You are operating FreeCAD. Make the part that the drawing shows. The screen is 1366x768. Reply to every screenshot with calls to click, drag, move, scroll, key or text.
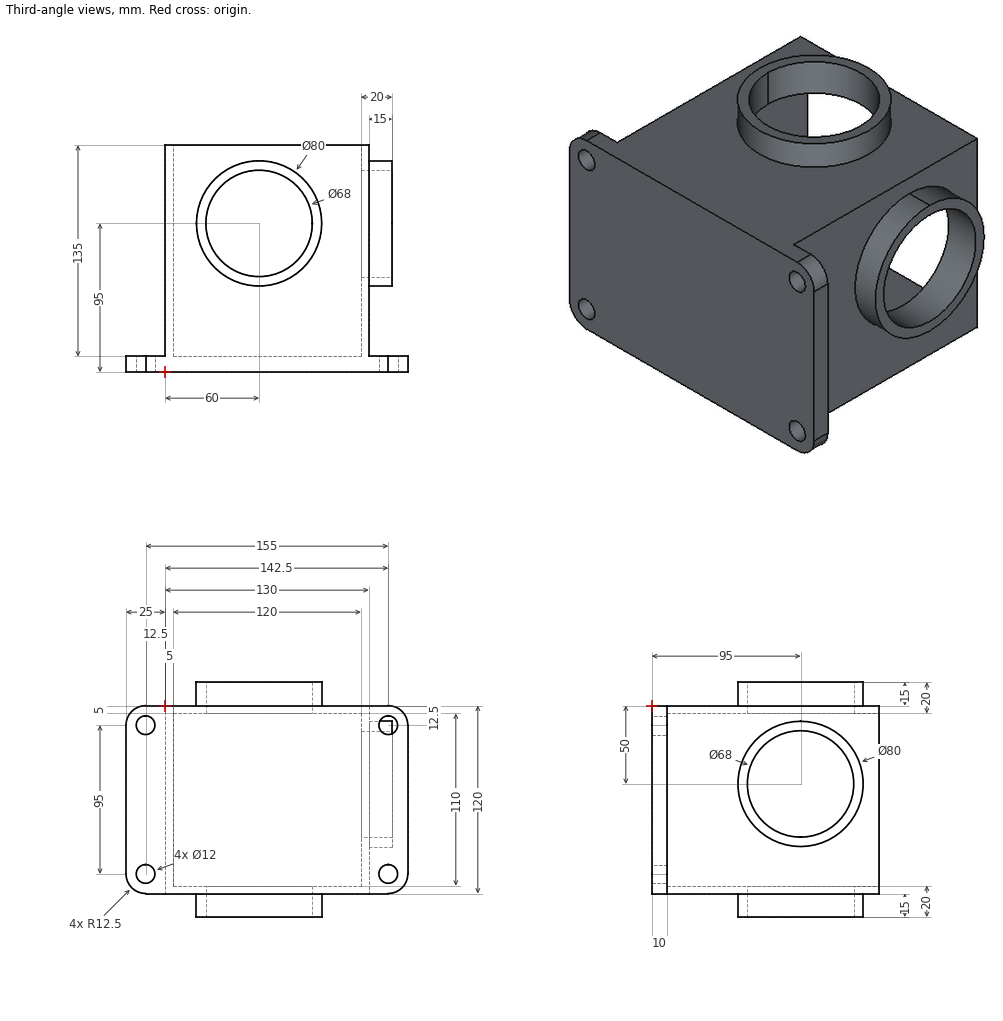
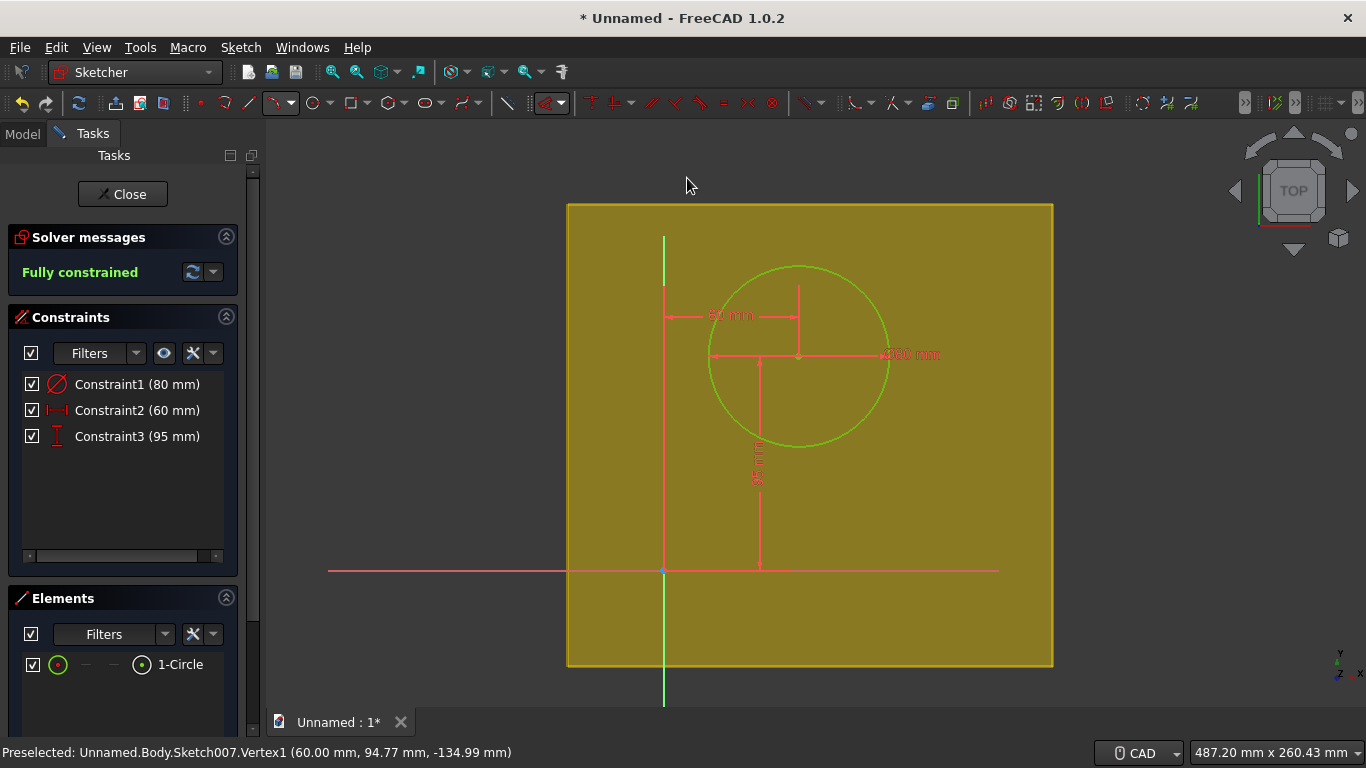
click(123, 194)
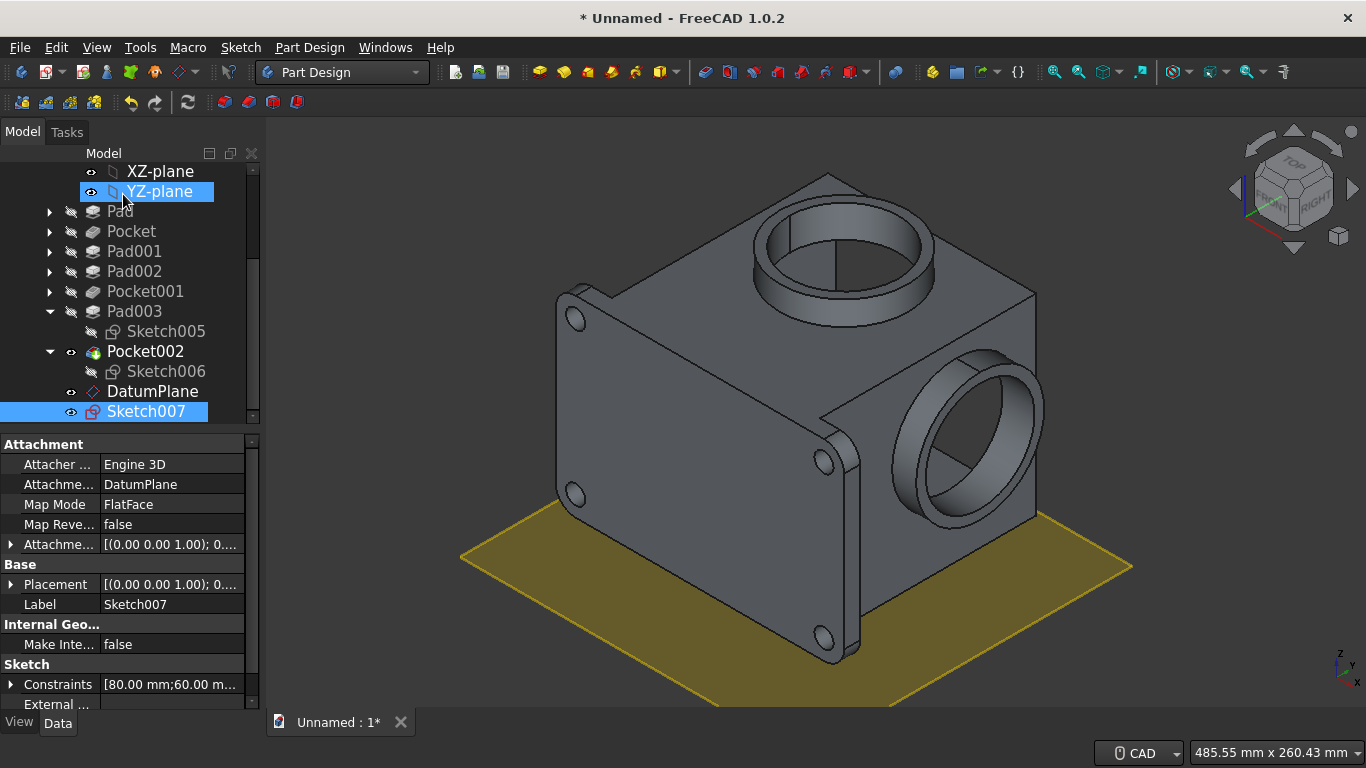
click(540, 72)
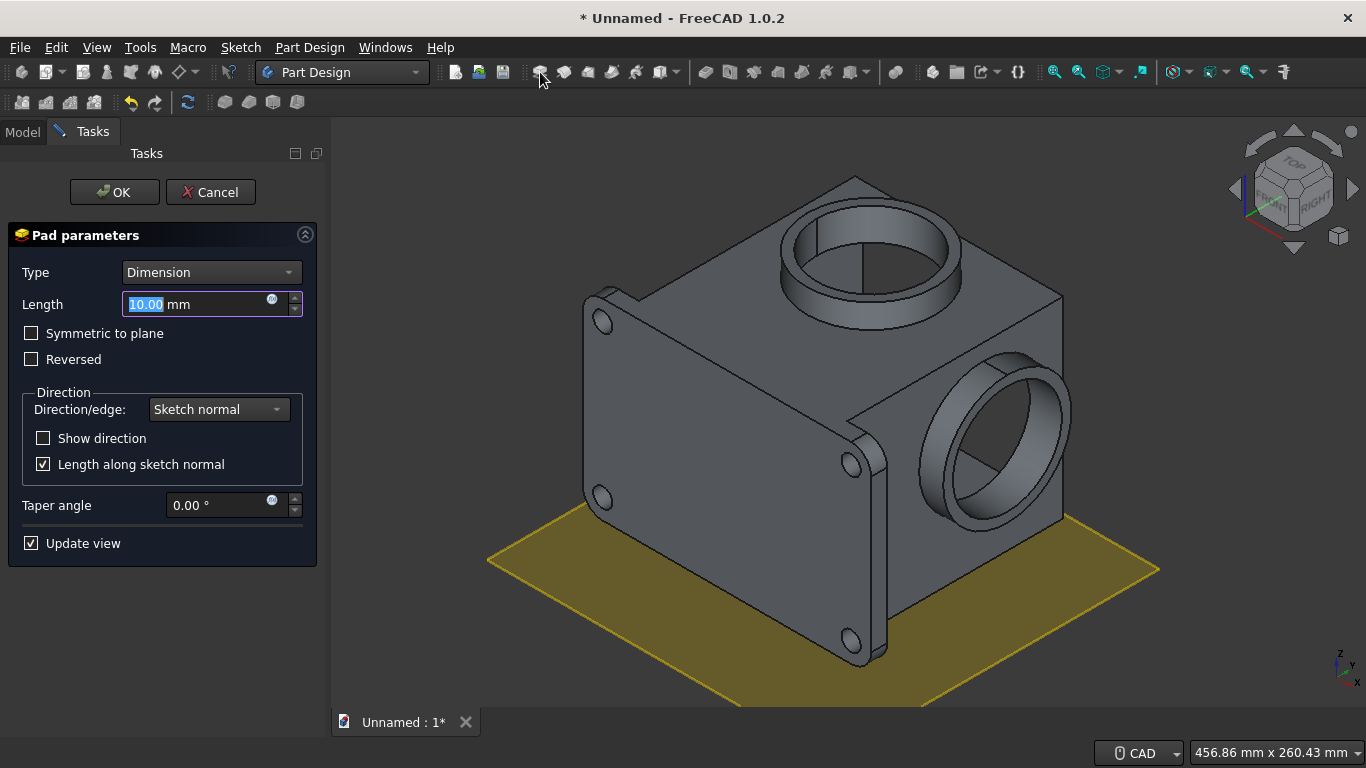
text(15)
key(Tab)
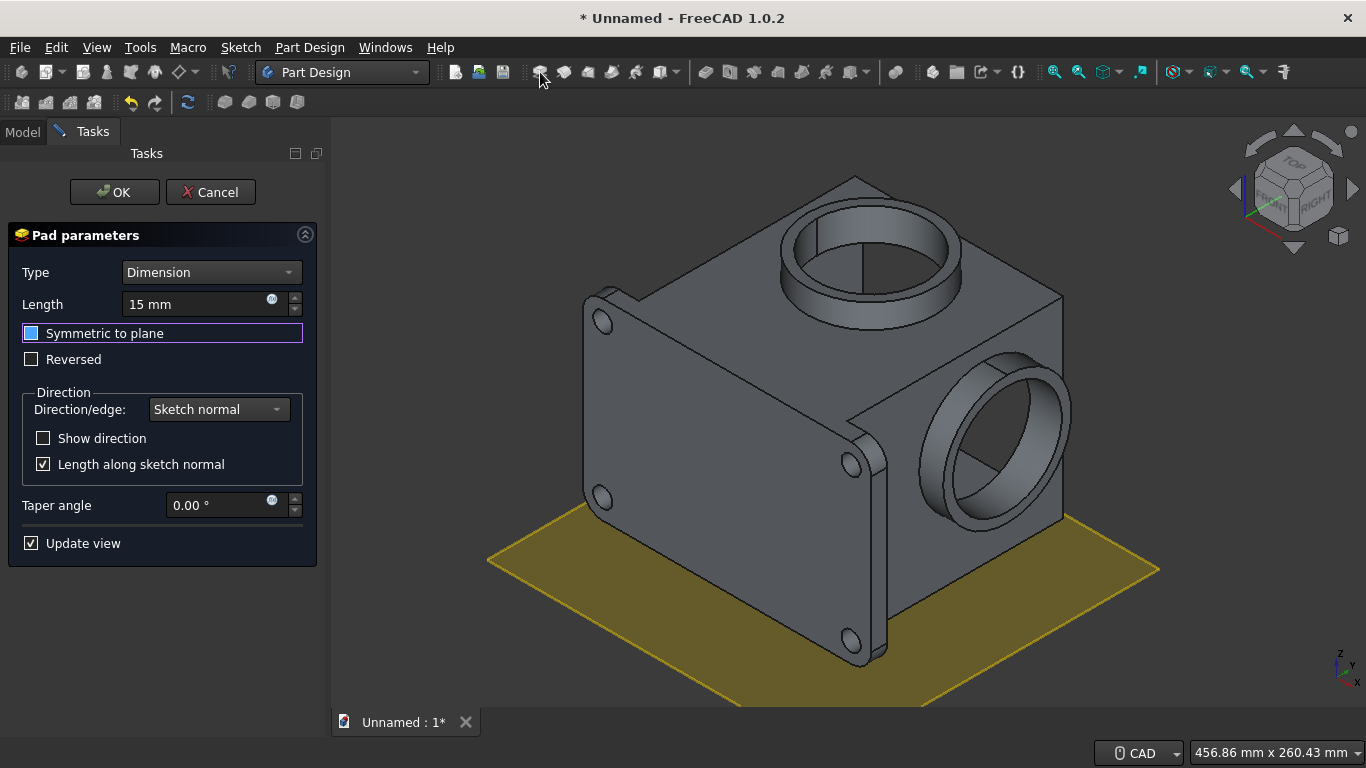
click(115, 192)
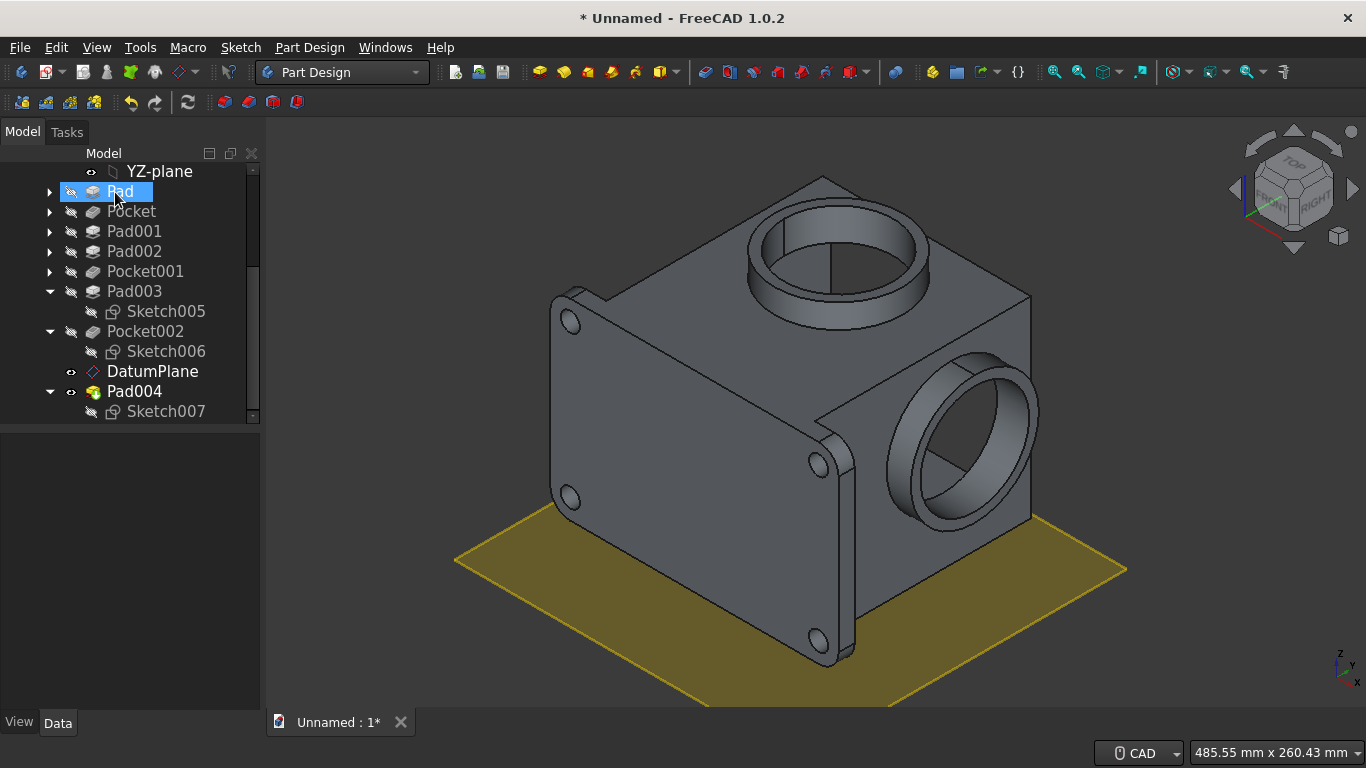
click(116, 372)
key(space)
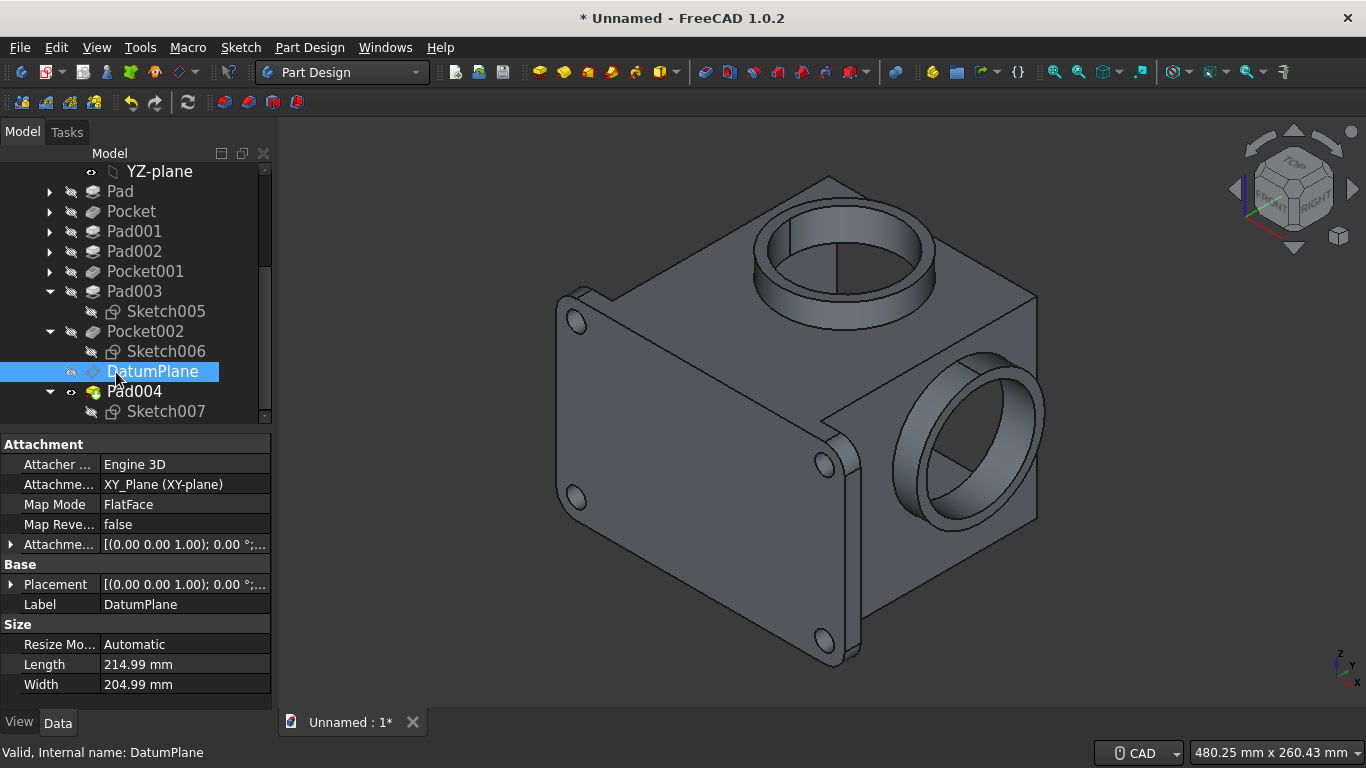
key(2)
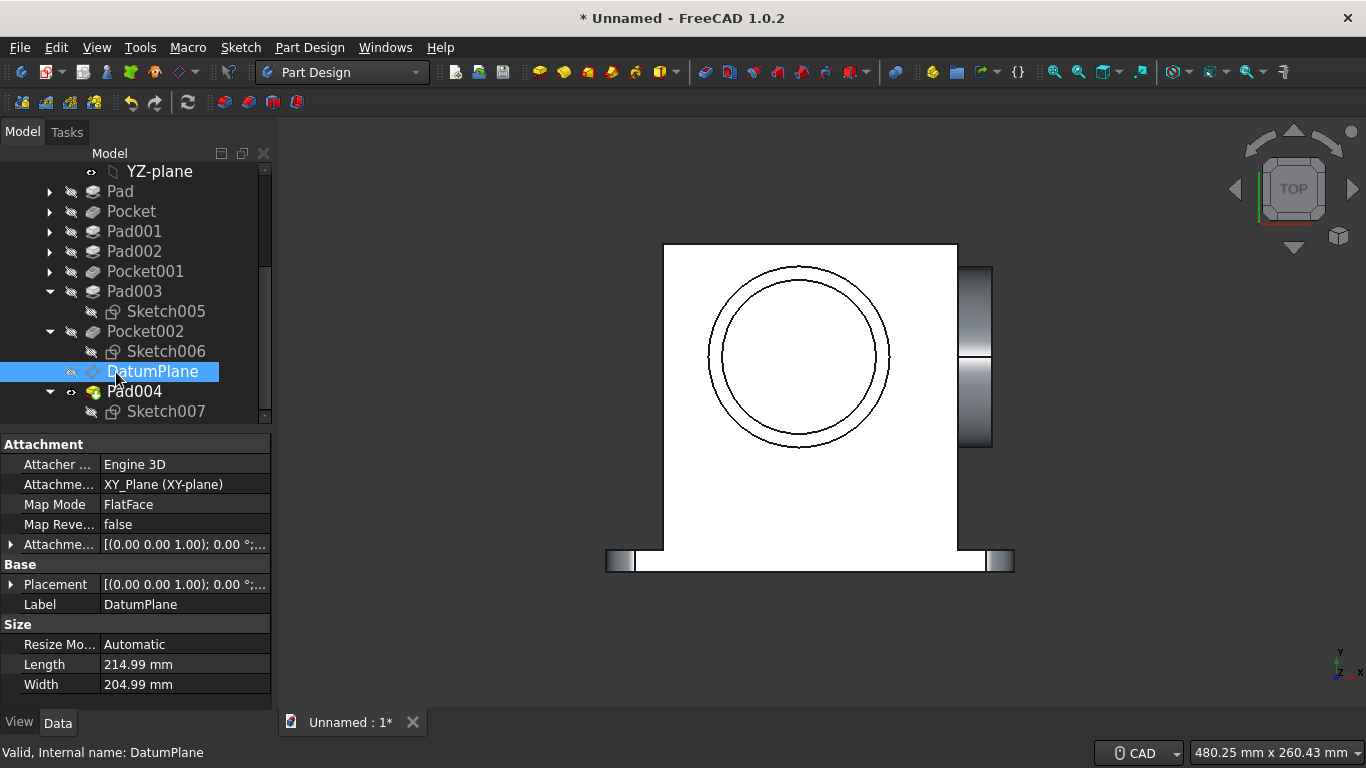
click(810, 396)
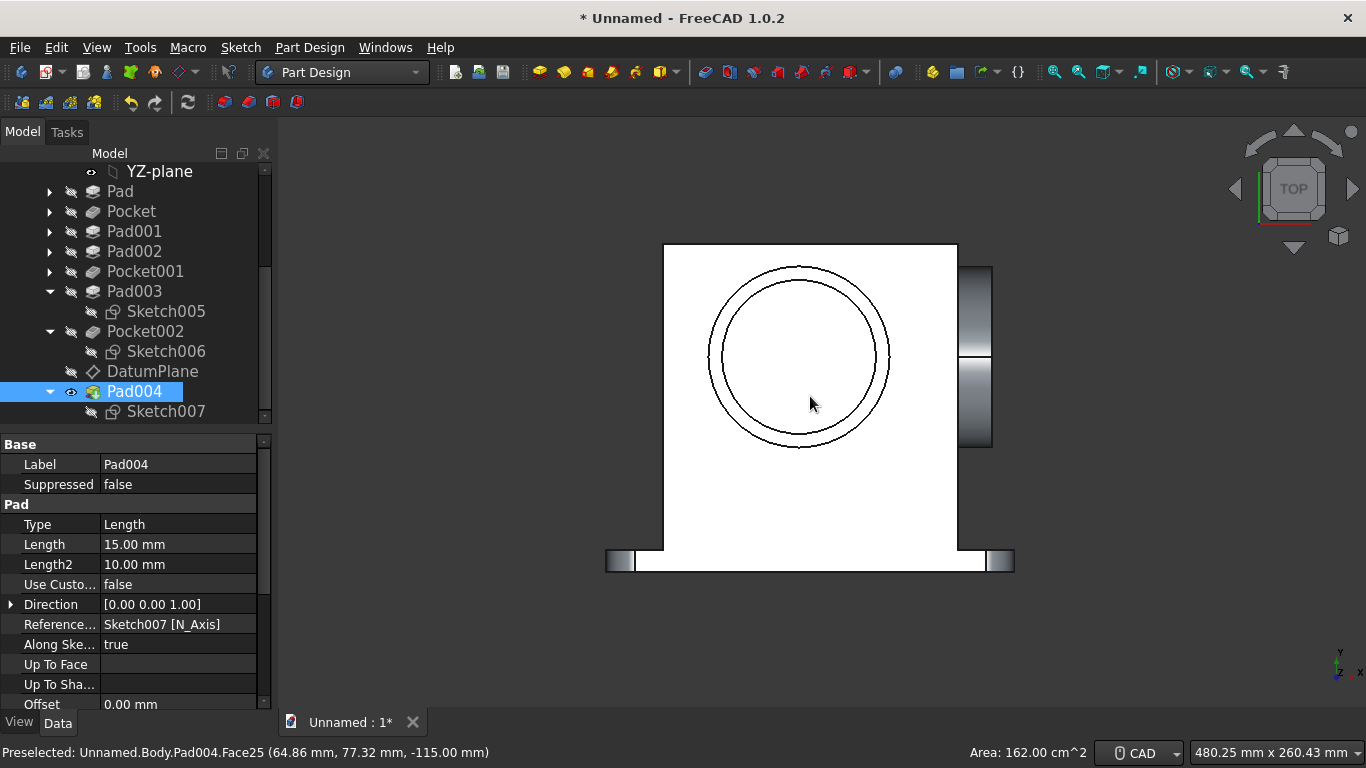
click(46, 72)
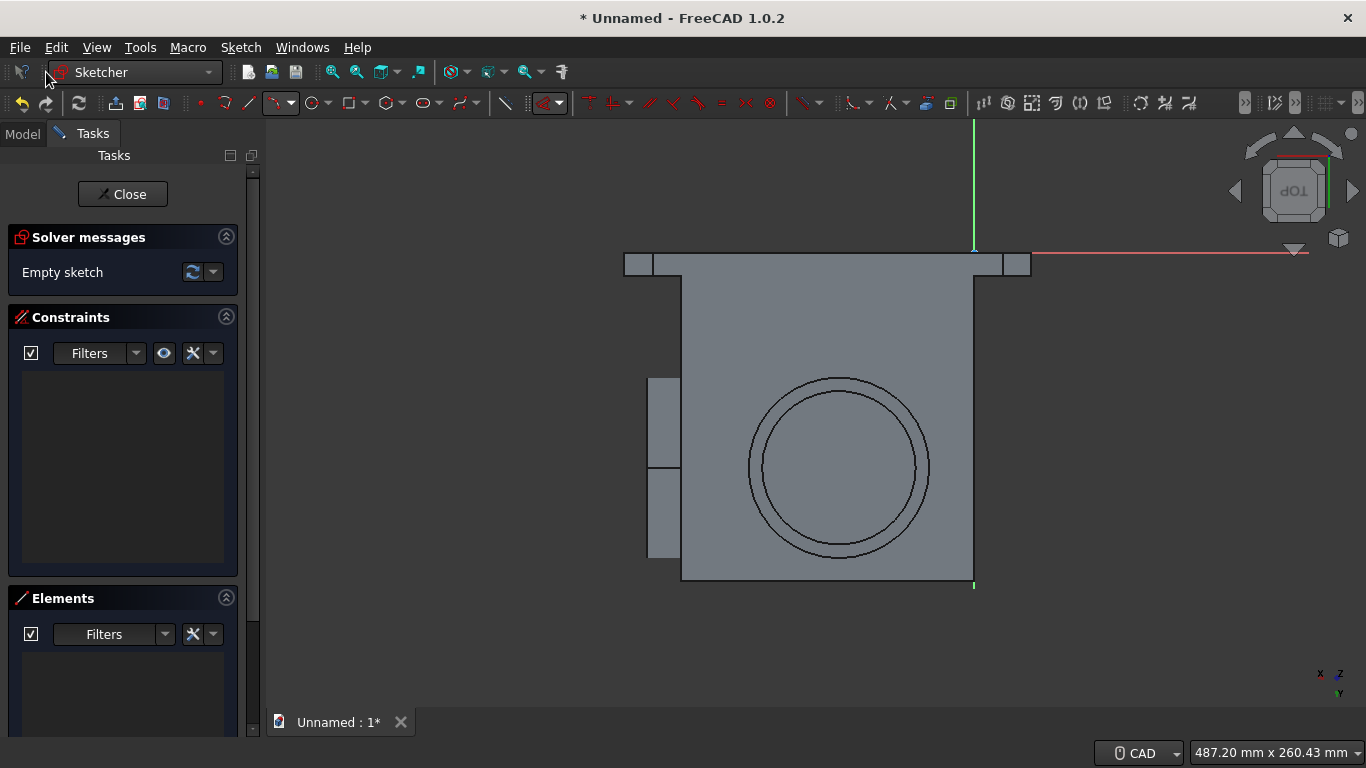
click(312, 104)